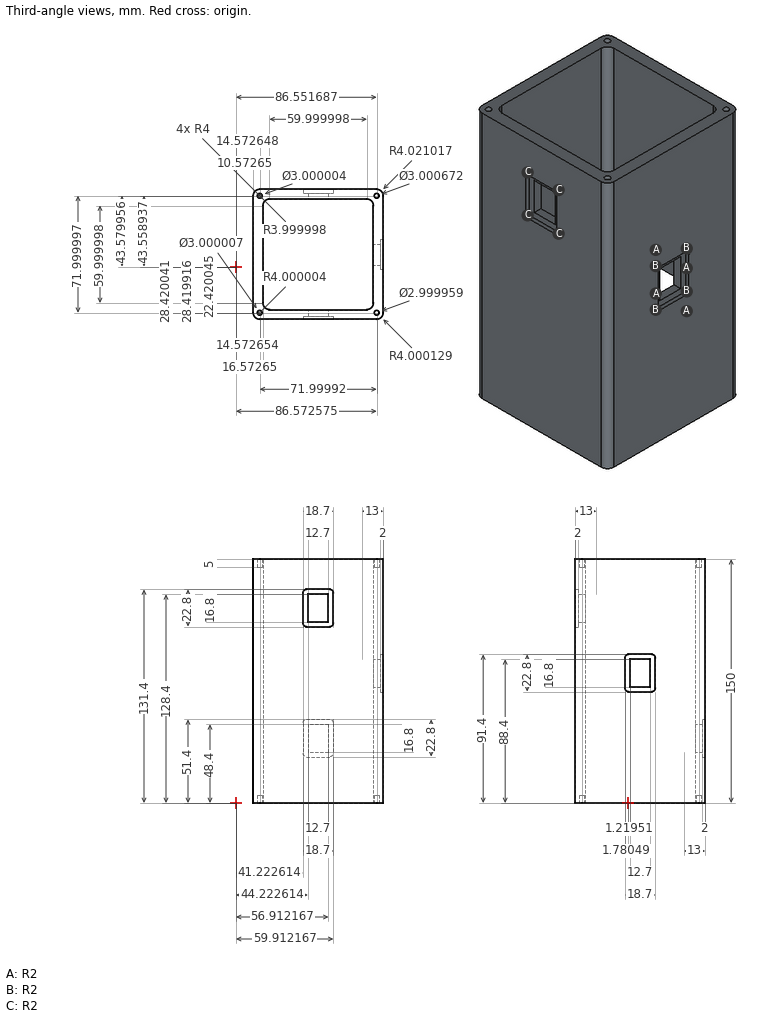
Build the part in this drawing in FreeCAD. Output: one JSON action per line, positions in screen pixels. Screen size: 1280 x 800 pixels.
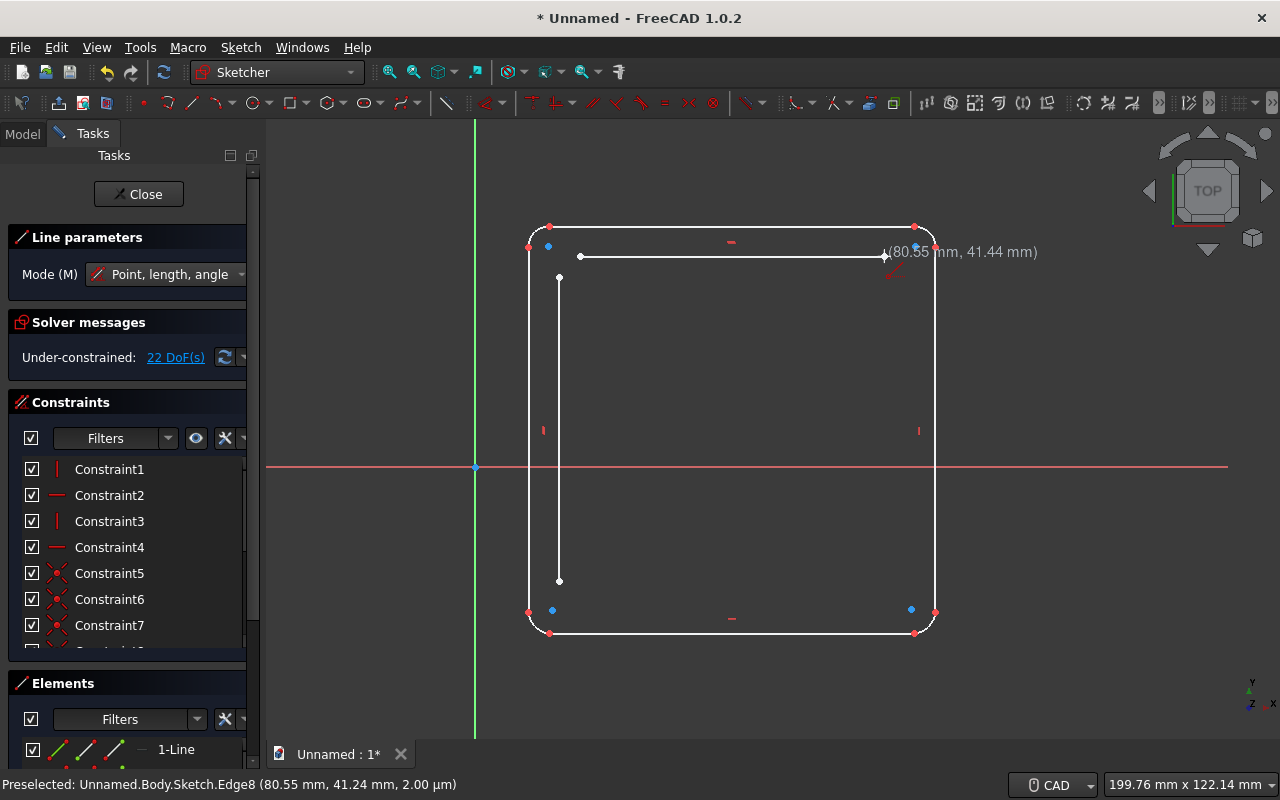
{"action": "left_click", "coordinate": [904, 277]}
{"action": "left_click", "coordinate": [904, 581]}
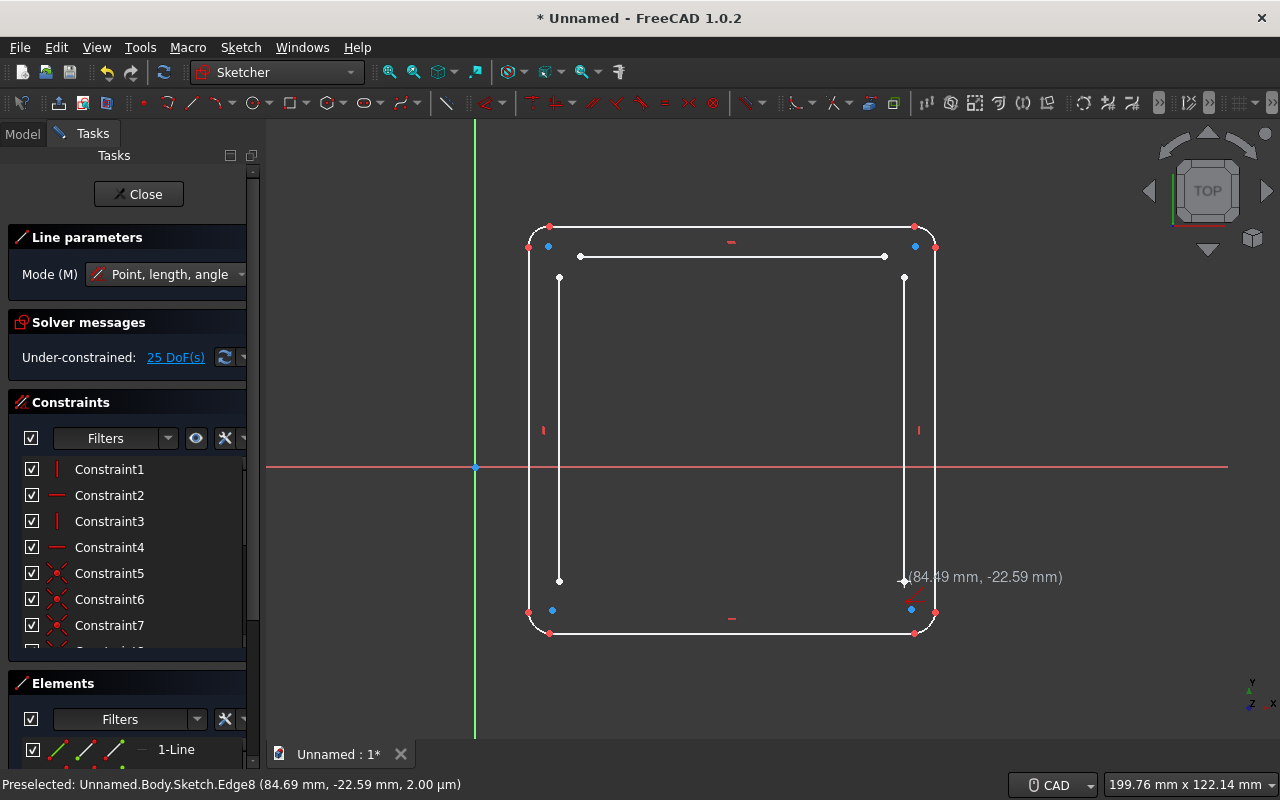
{"action": "left_click", "coordinate": [884, 601]}
{"action": "left_click", "coordinate": [580, 601]}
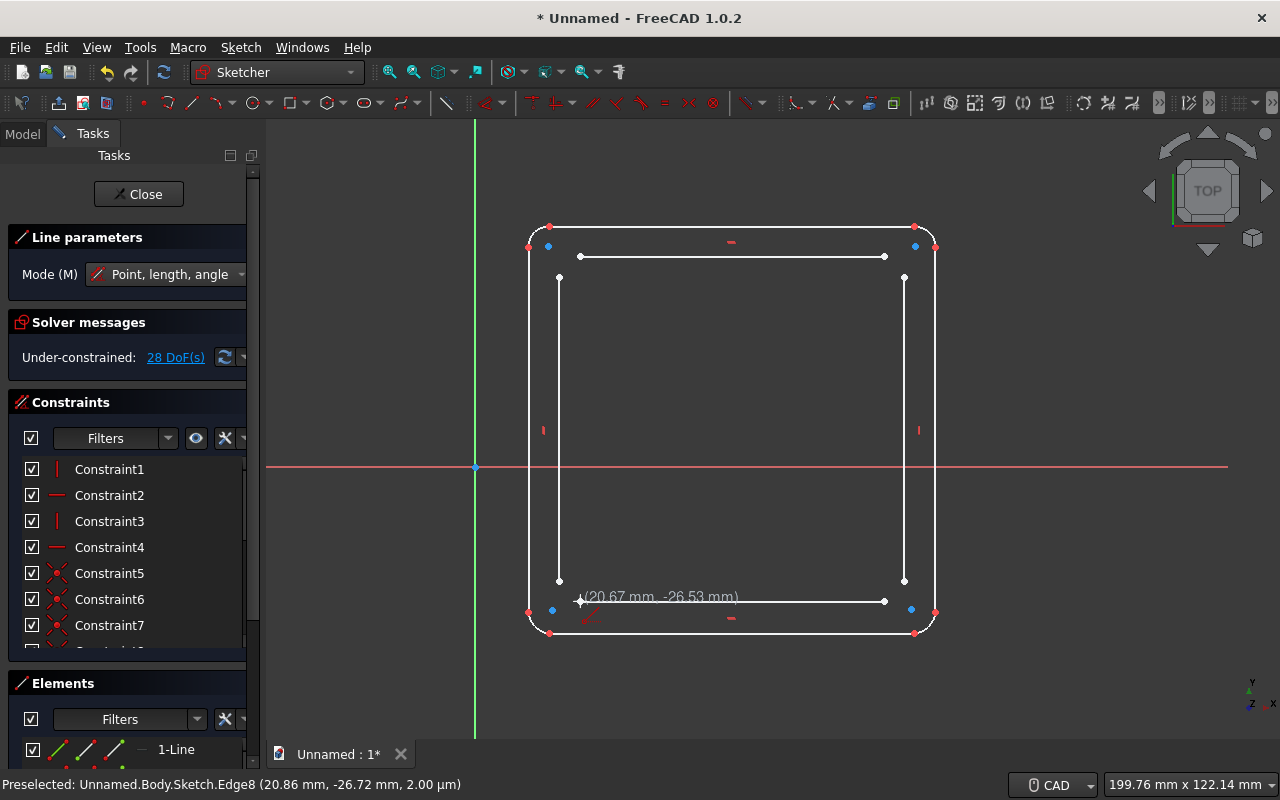
{"action": "left_click", "coordinate": [216, 104]}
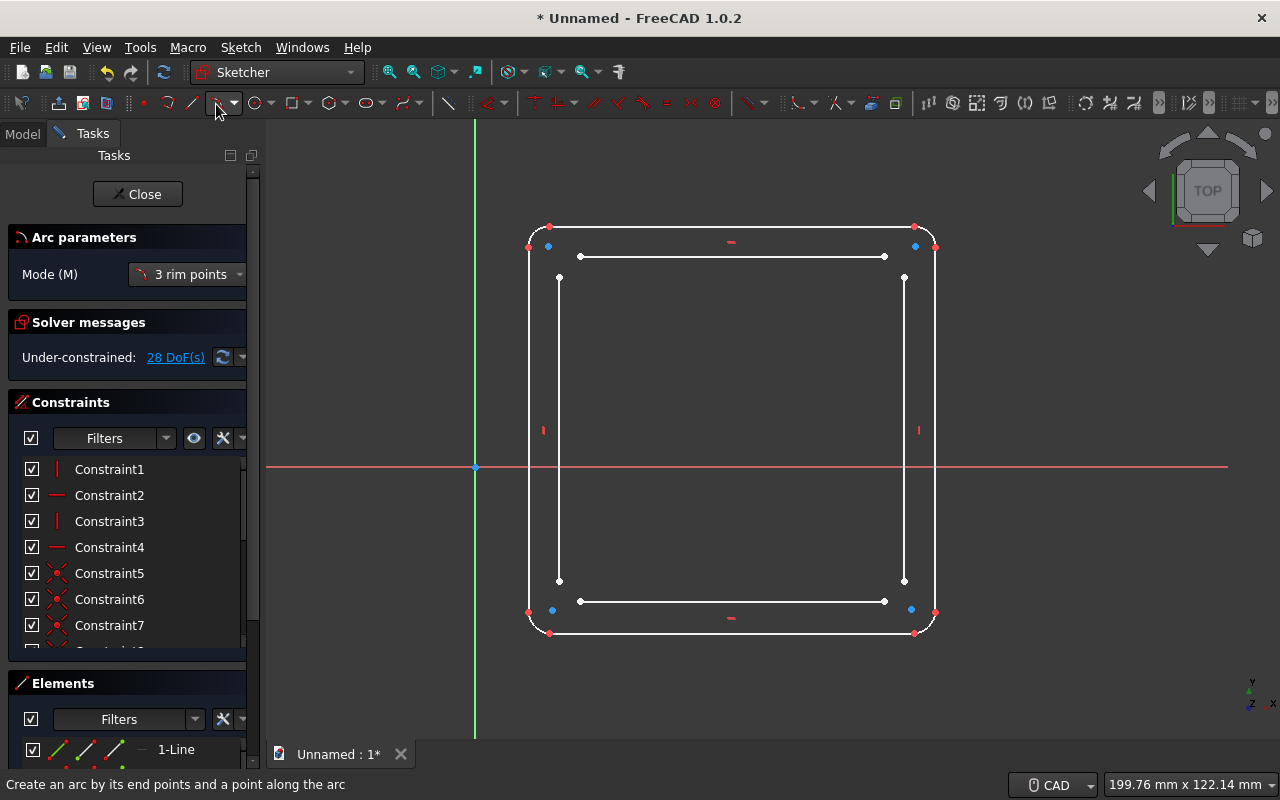
{"action": "left_click", "coordinate": [559, 278]}
{"action": "left_click", "coordinate": [580, 257]}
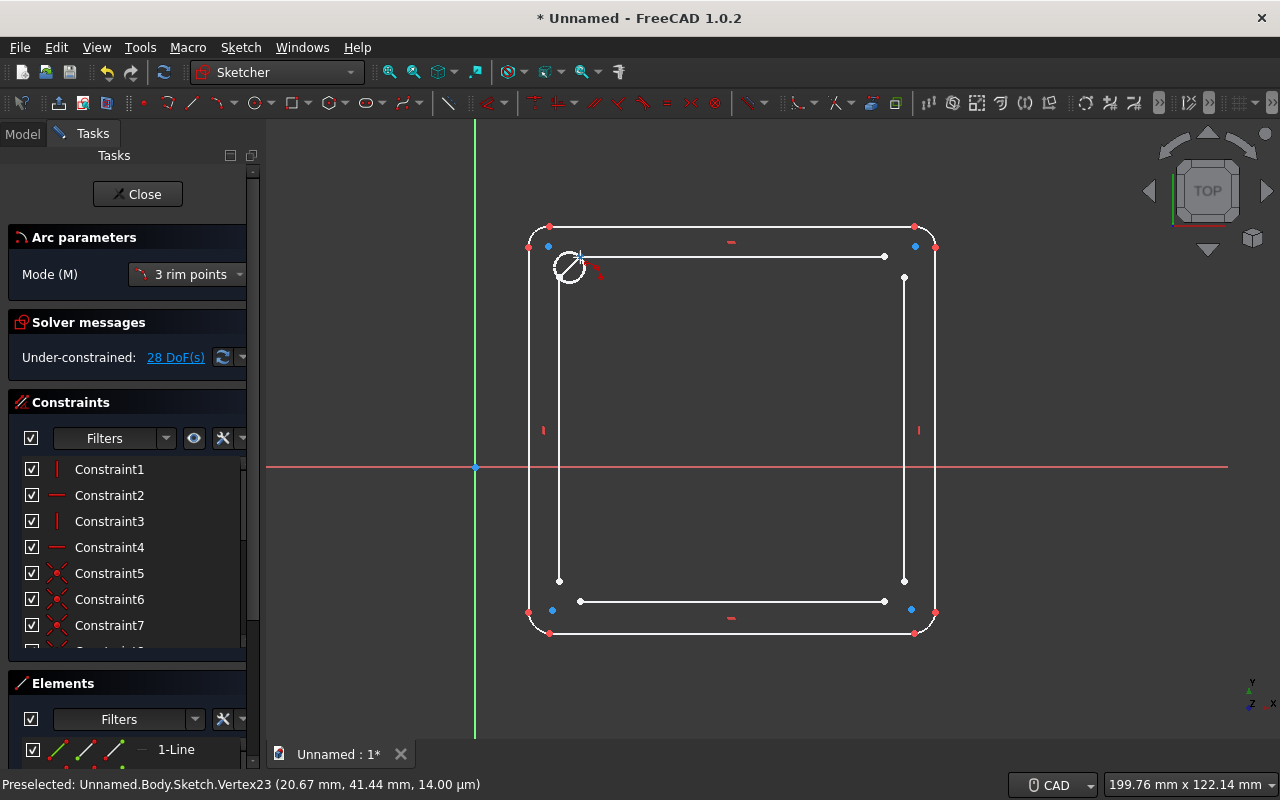
{"action": "scroll", "coordinate": [565, 262], "scroll_direction": "up", "scroll_amount": 5}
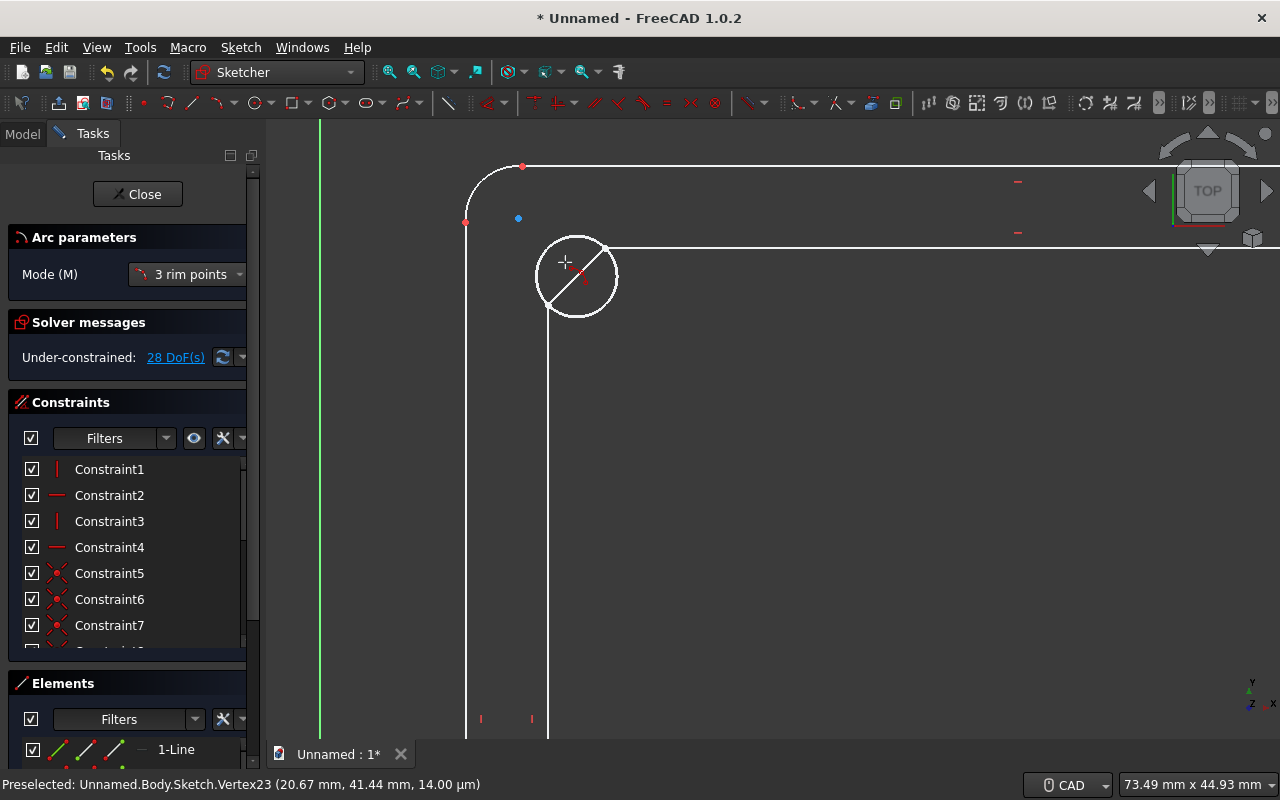
{"action": "left_click", "coordinate": [565, 262]}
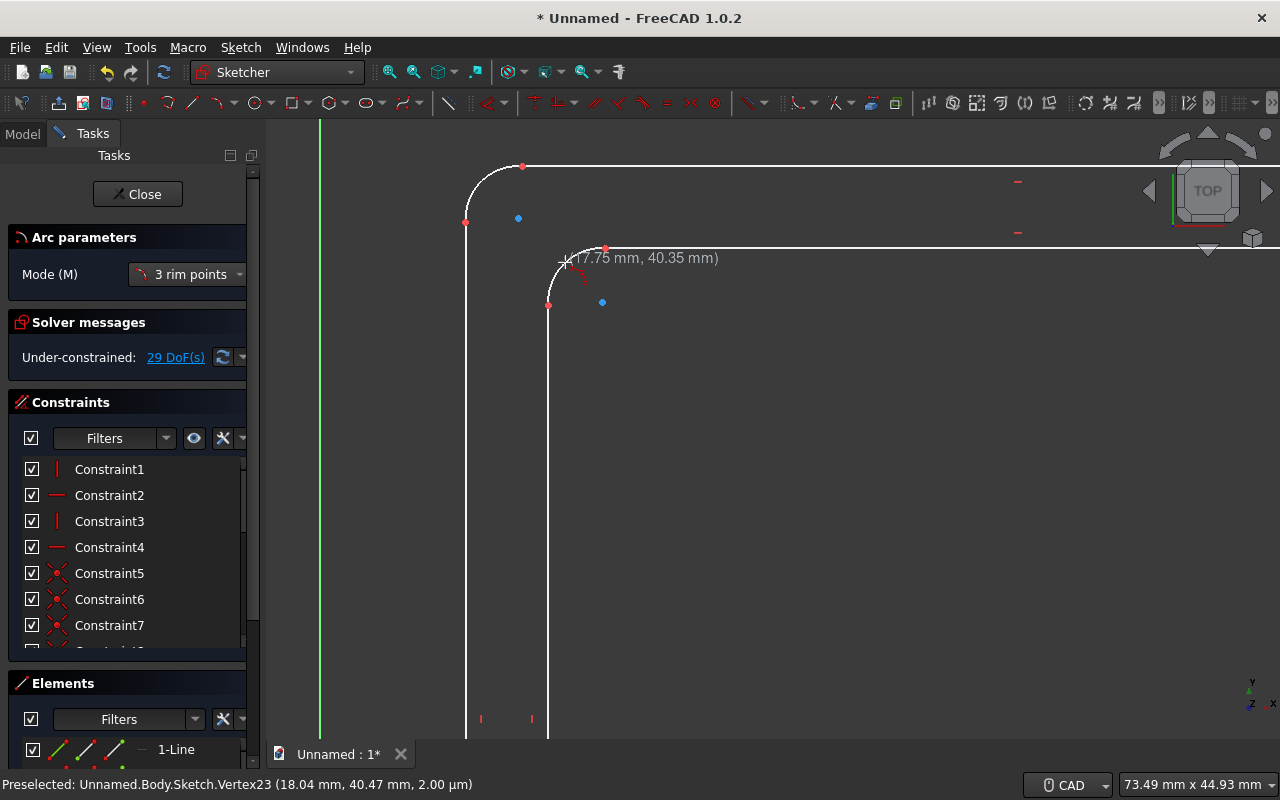
{"action": "scroll", "coordinate": [565, 262], "scroll_direction": "down", "scroll_amount": 5}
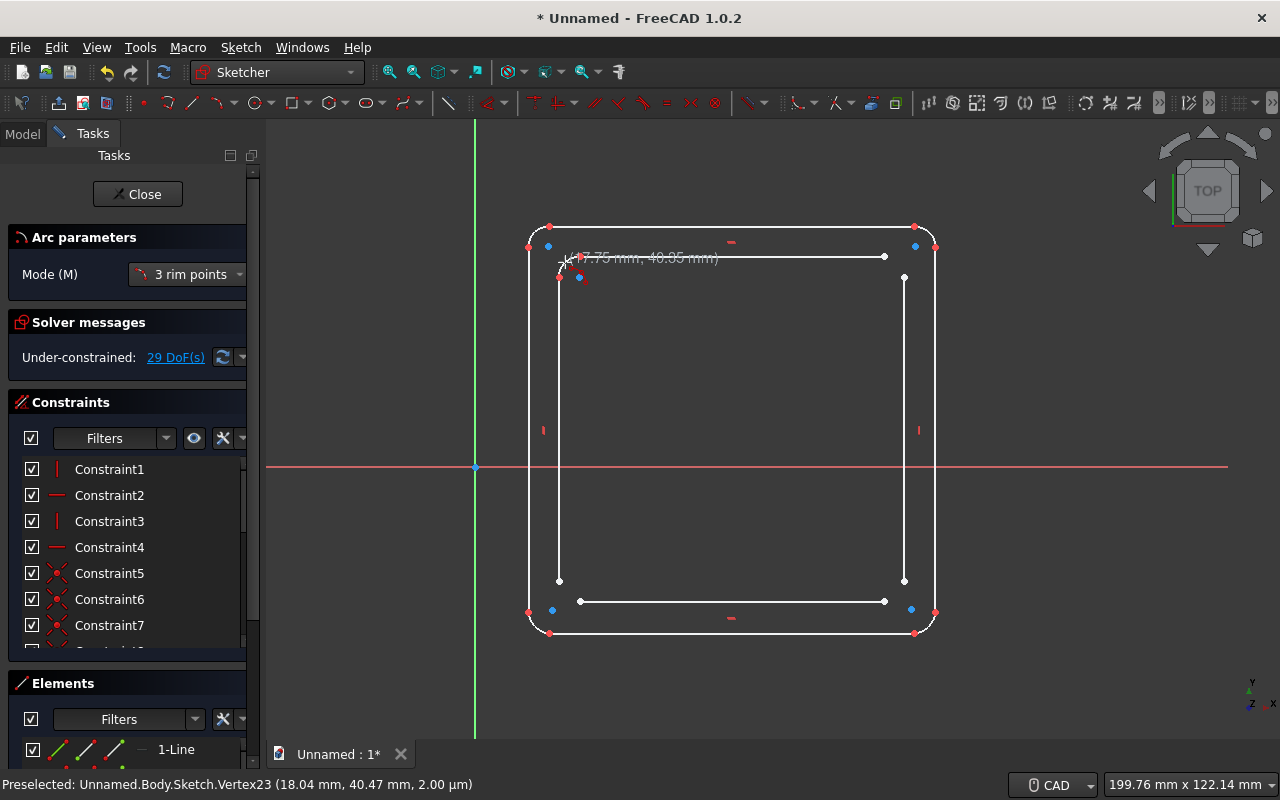
{"action": "left_click", "coordinate": [884, 257]}
{"action": "left_click", "coordinate": [904, 278]}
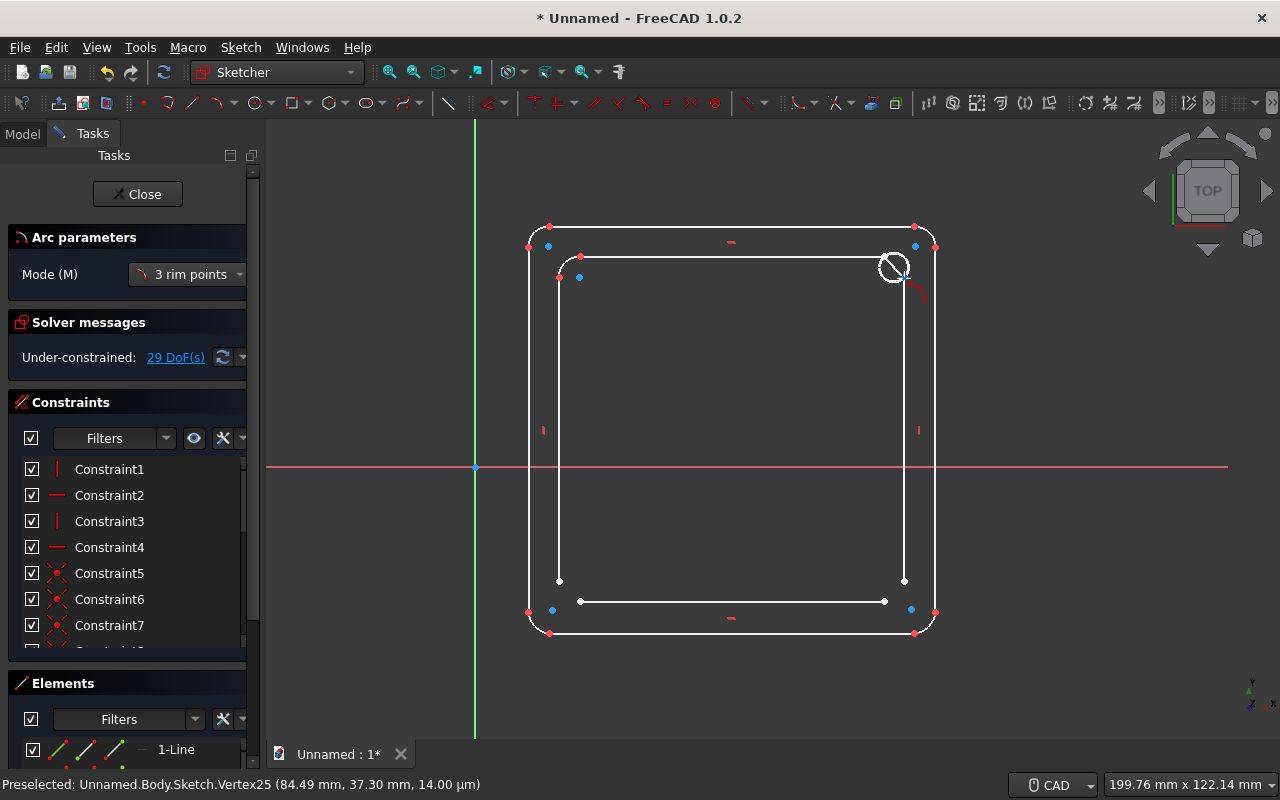
{"action": "scroll", "coordinate": [898, 262], "scroll_direction": "up", "scroll_amount": 5}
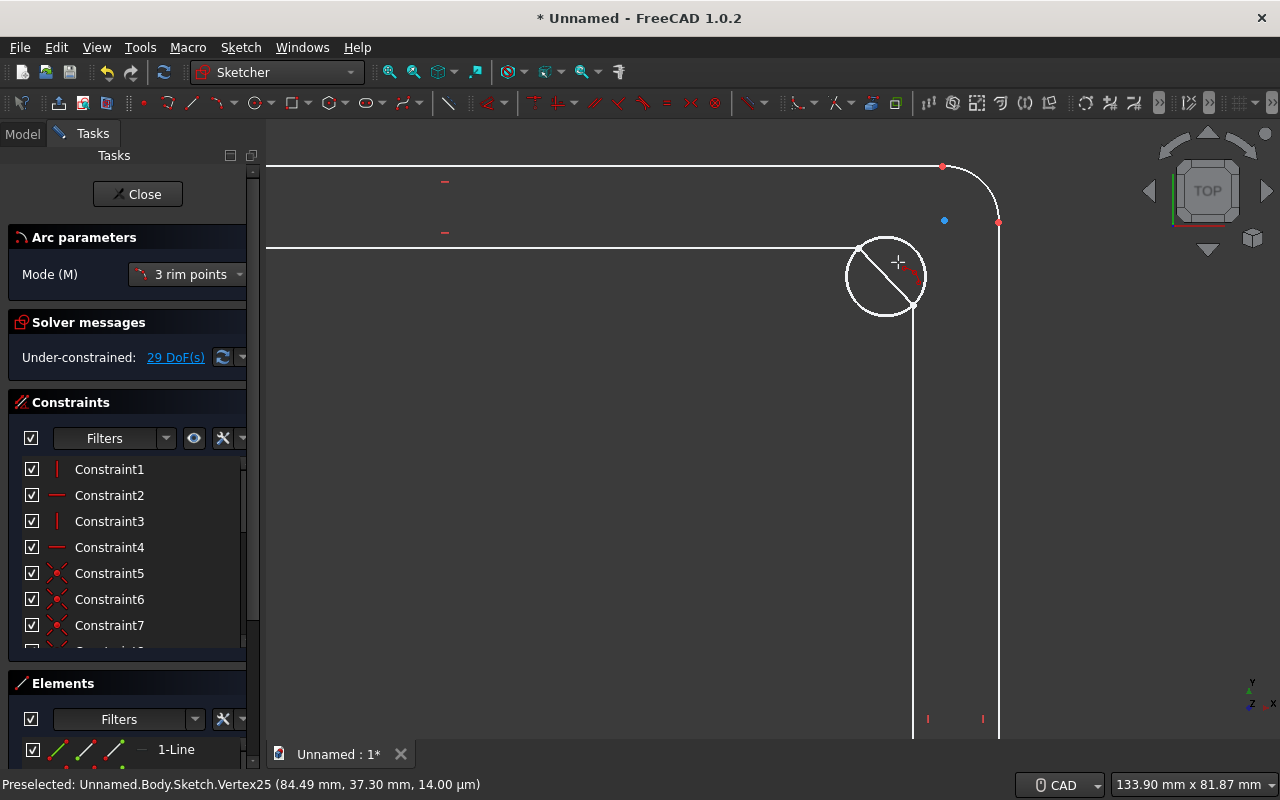
{"action": "left_click", "coordinate": [898, 262]}